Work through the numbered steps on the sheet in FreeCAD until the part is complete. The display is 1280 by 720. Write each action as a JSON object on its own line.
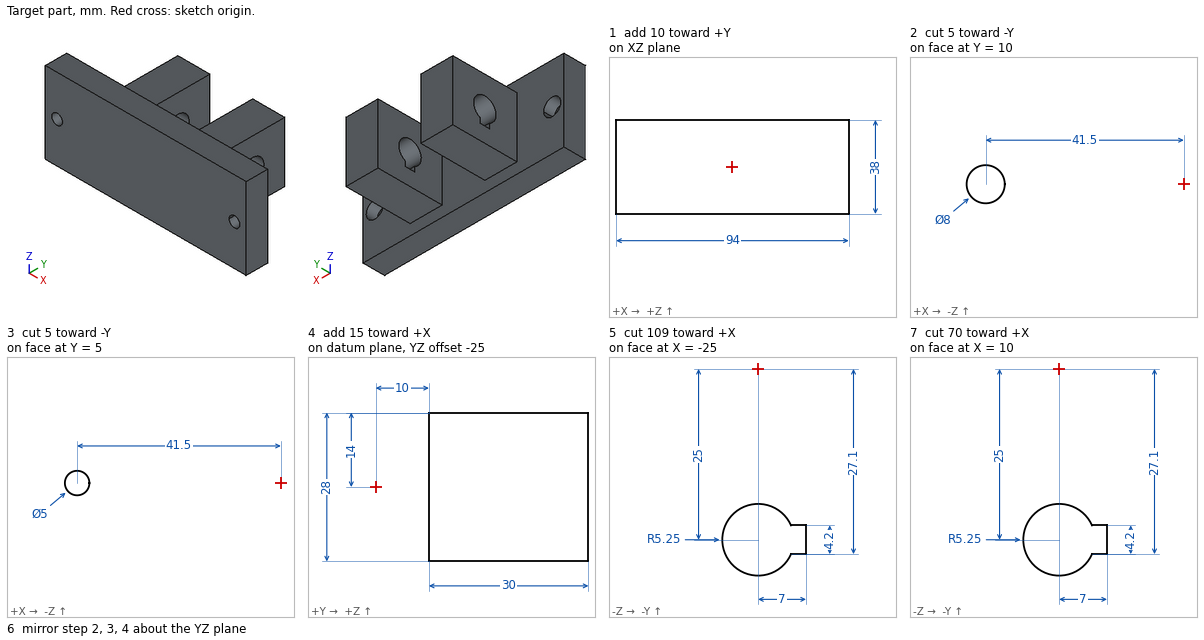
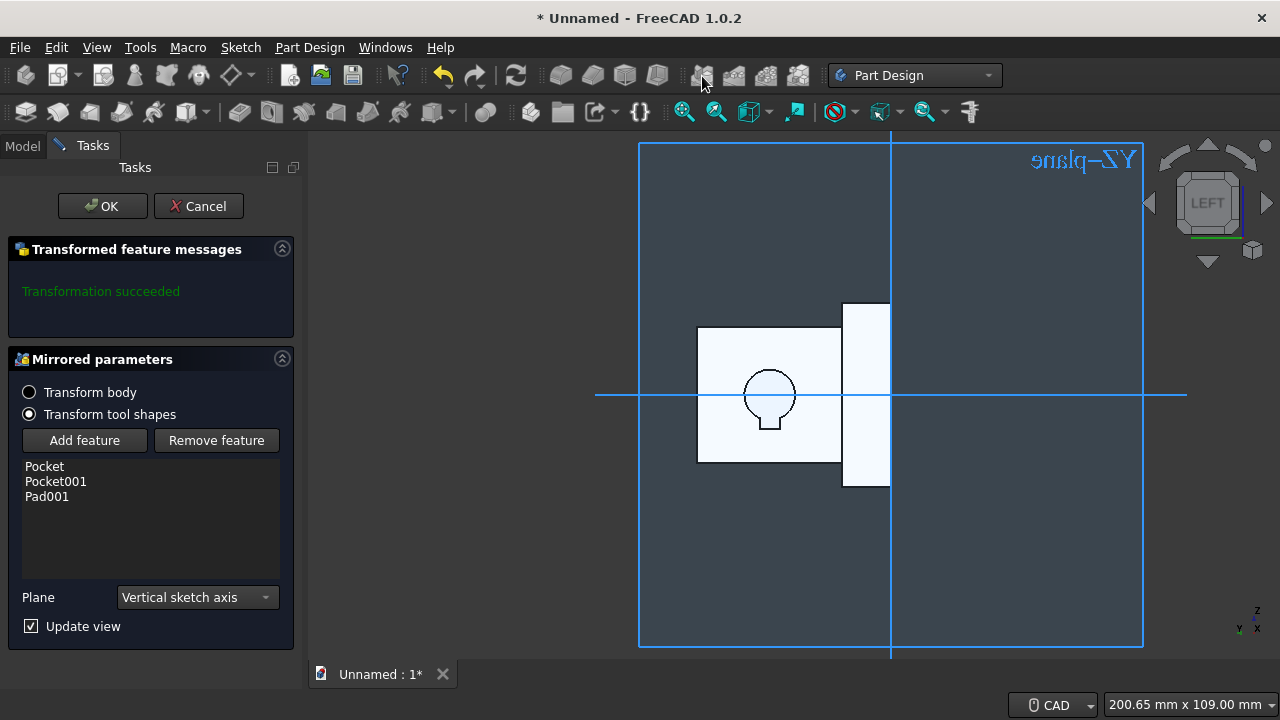
{"action": "left_click", "coordinate": [198, 598]}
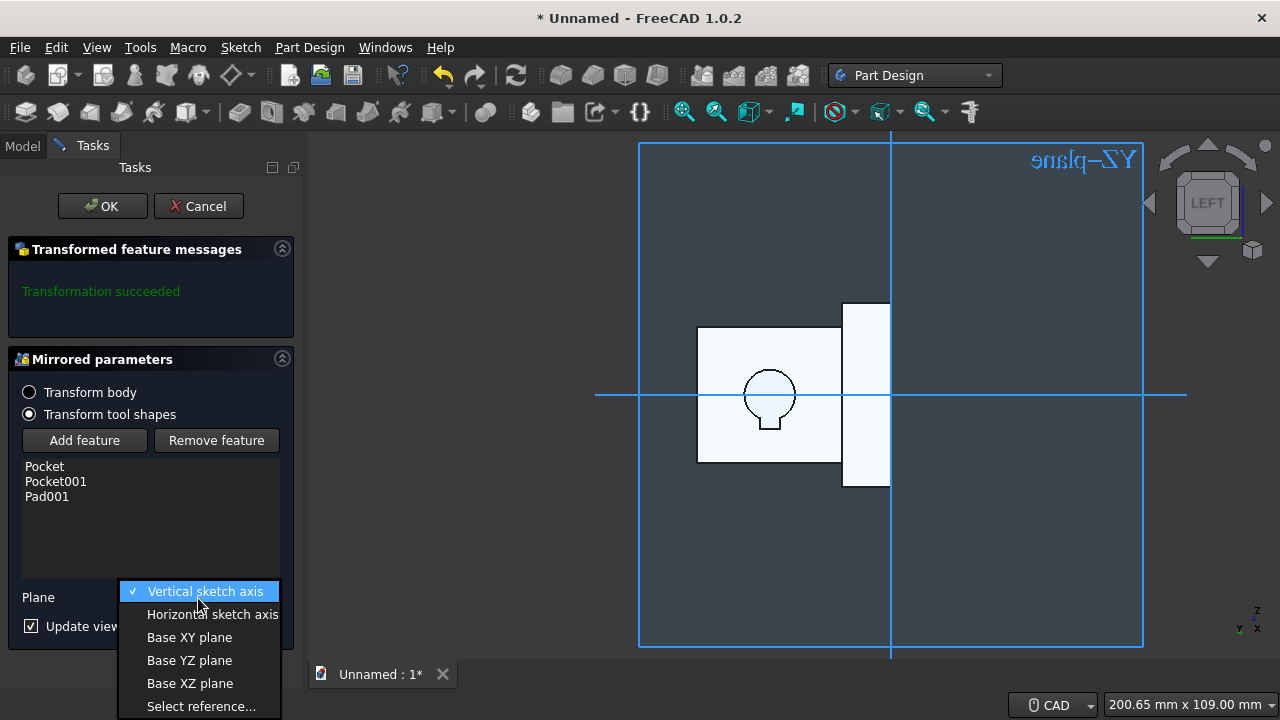
{"action": "left_click", "coordinate": [198, 660]}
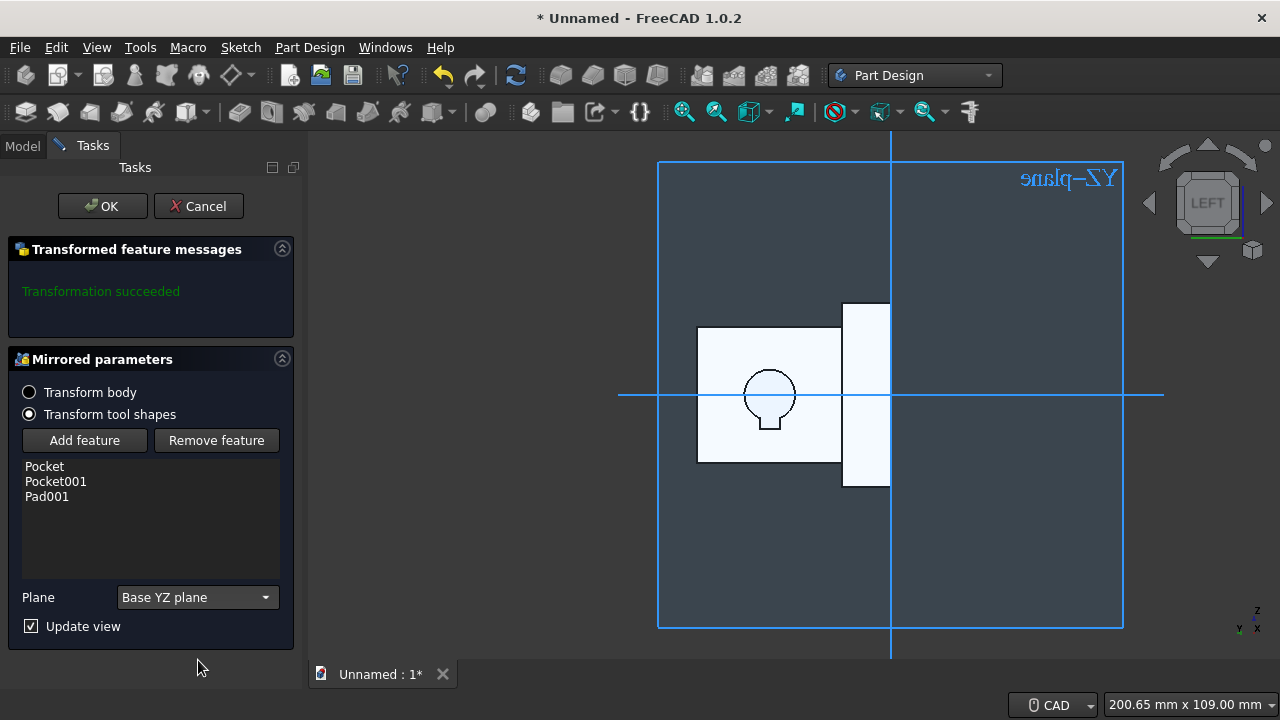
{"action": "left_click", "coordinate": [103, 206]}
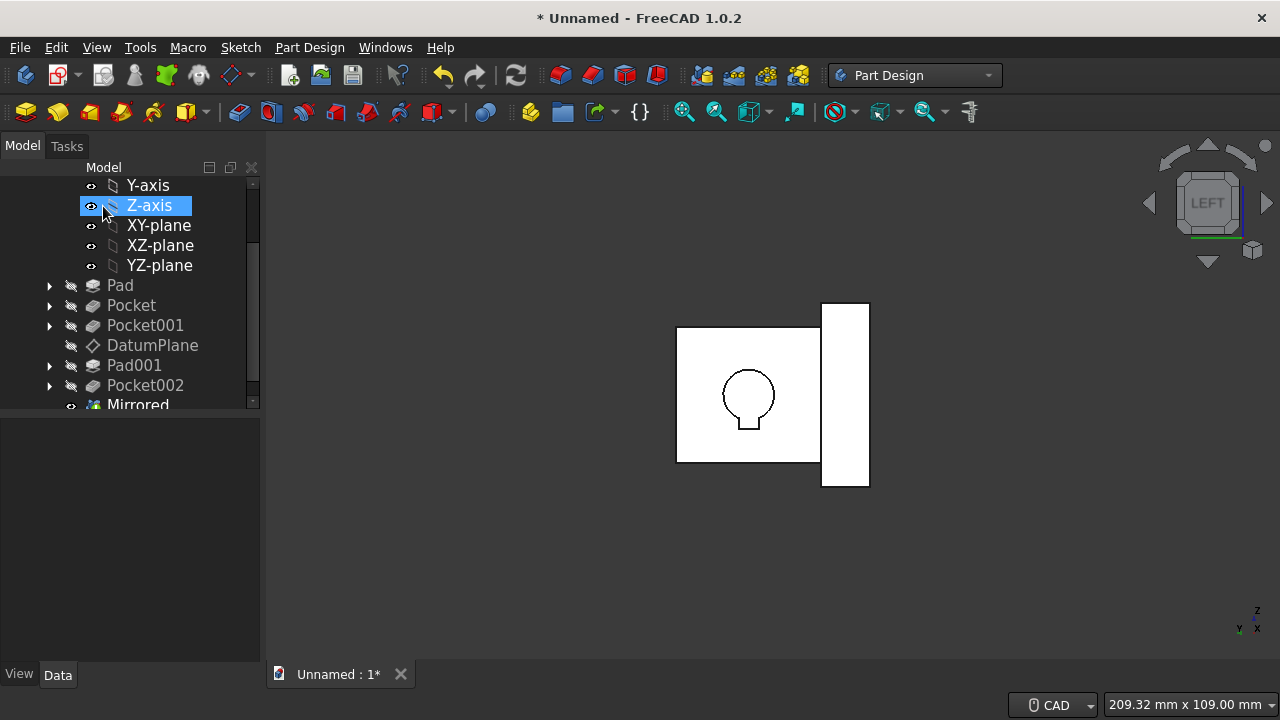
{"action": "left_click", "coordinate": [686, 112]}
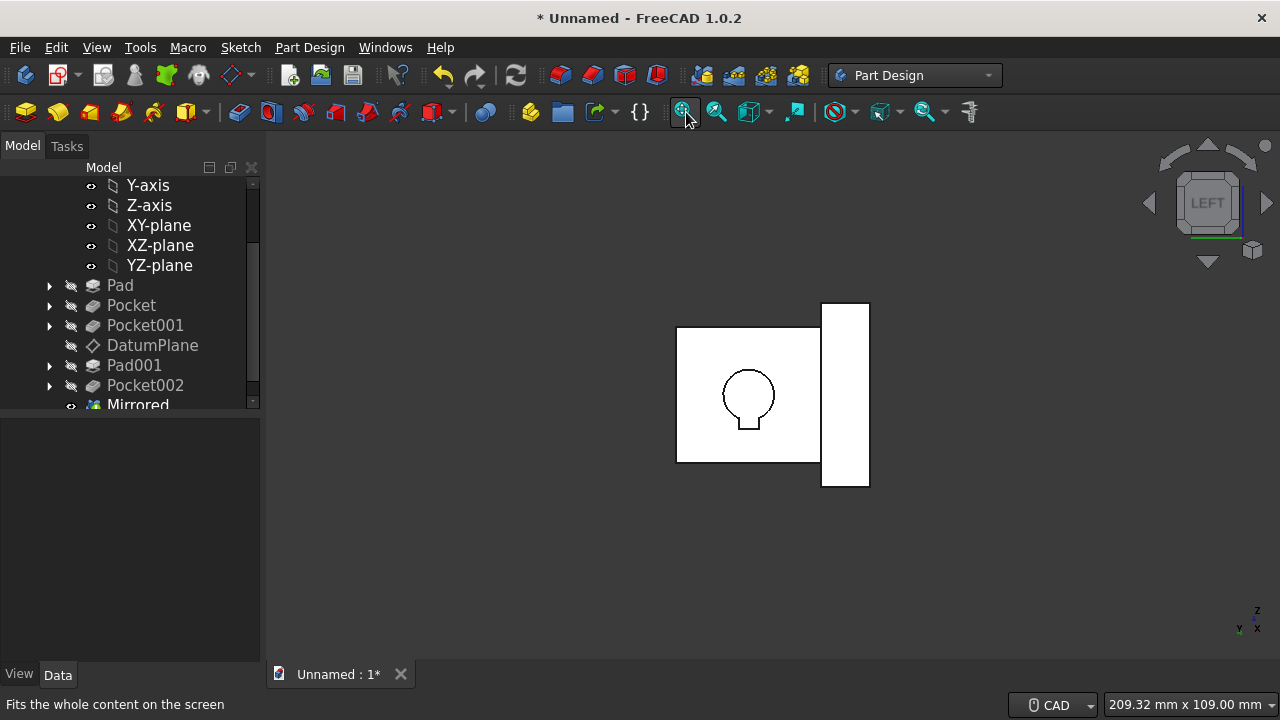
{"action": "left_click", "coordinate": [749, 394]}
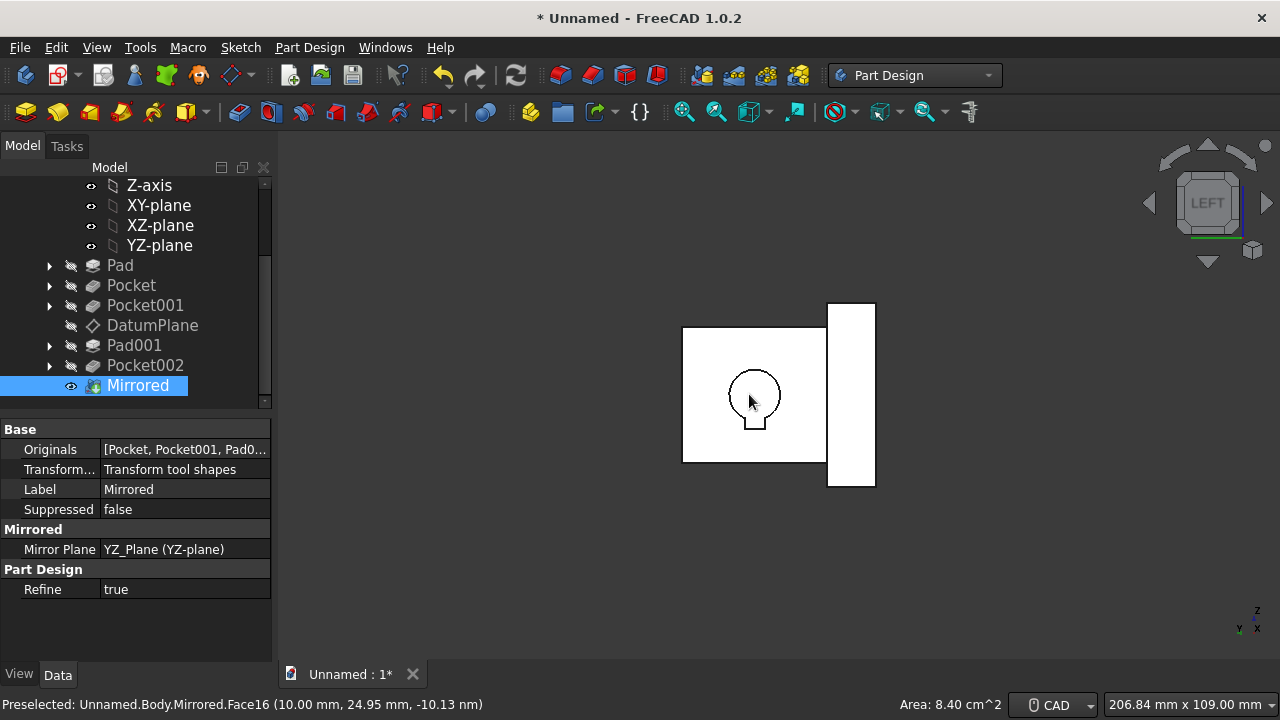
{"action": "left_click", "coordinate": [58, 76]}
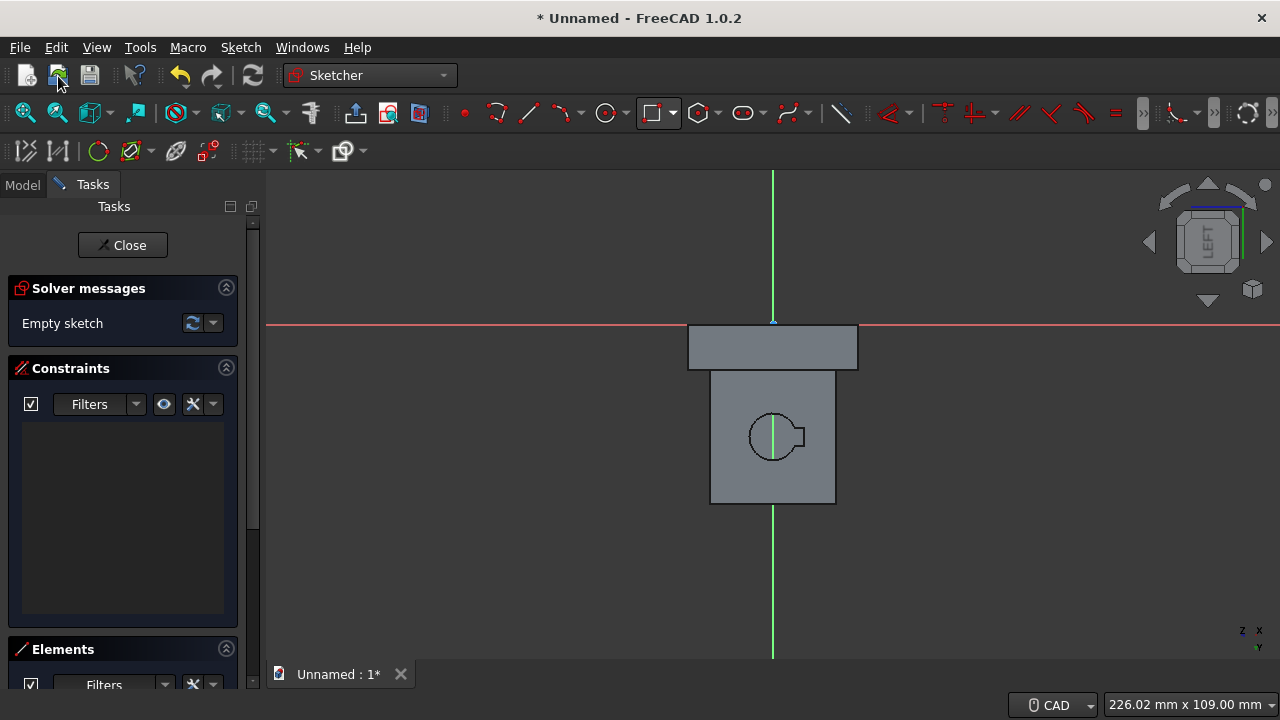
{"action": "scroll", "coordinate": [819, 369], "scroll_direction": "up", "scroll_amount": 5}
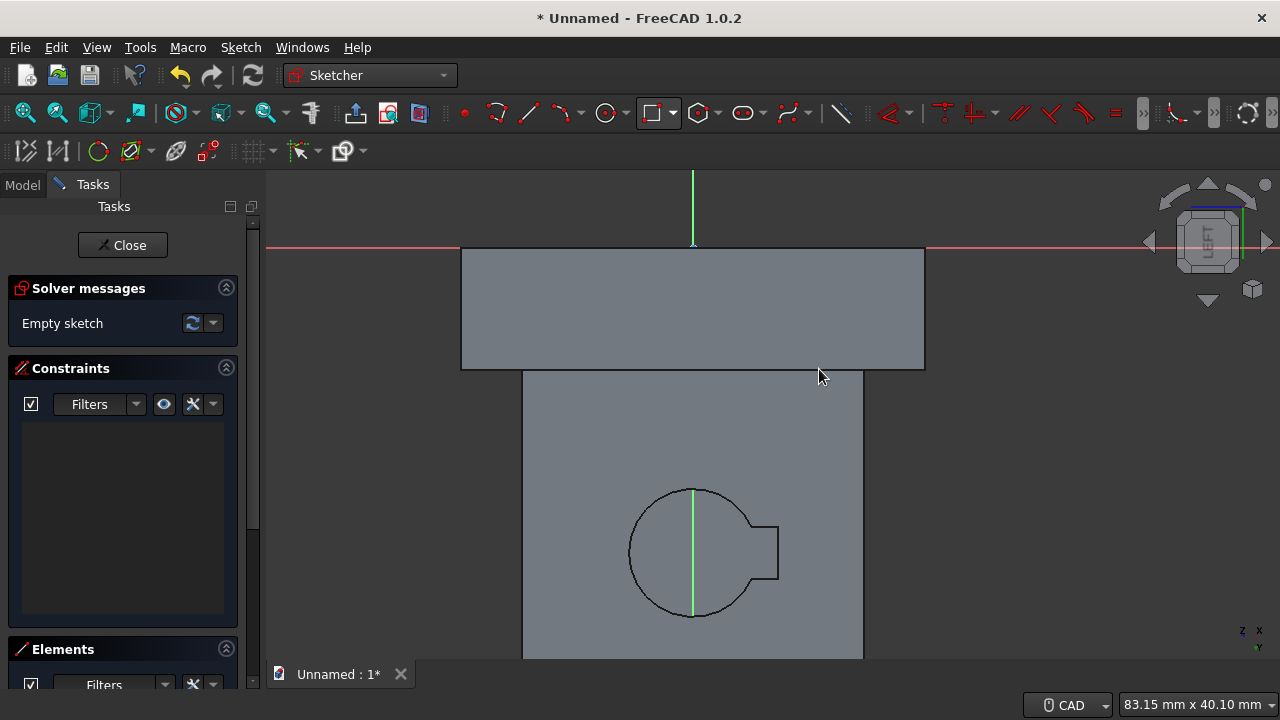
{"action": "left_click", "coordinate": [498, 114]}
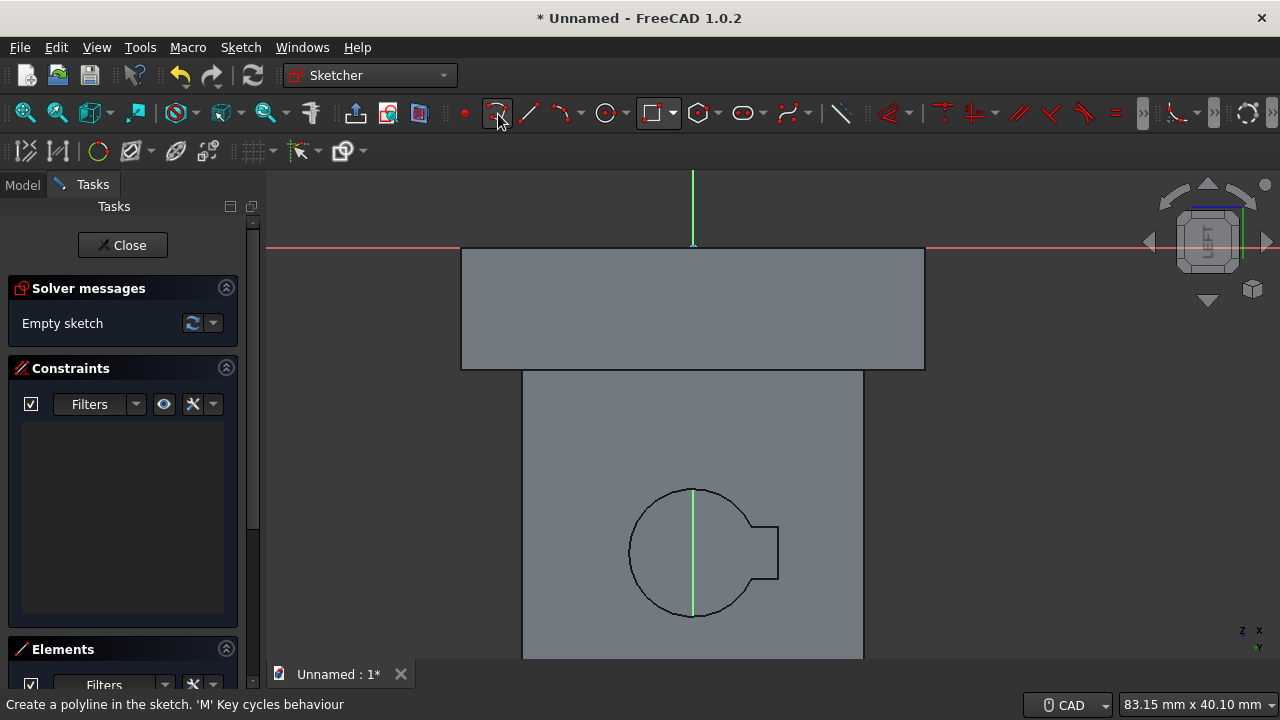
{"action": "left_click", "coordinate": [752, 579]}
{"action": "left_click", "coordinate": [778, 579]}
{"action": "left_click", "coordinate": [778, 527]}
{"action": "left_click", "coordinate": [752, 527]}
{"action": "right_click", "coordinate": [752, 527]}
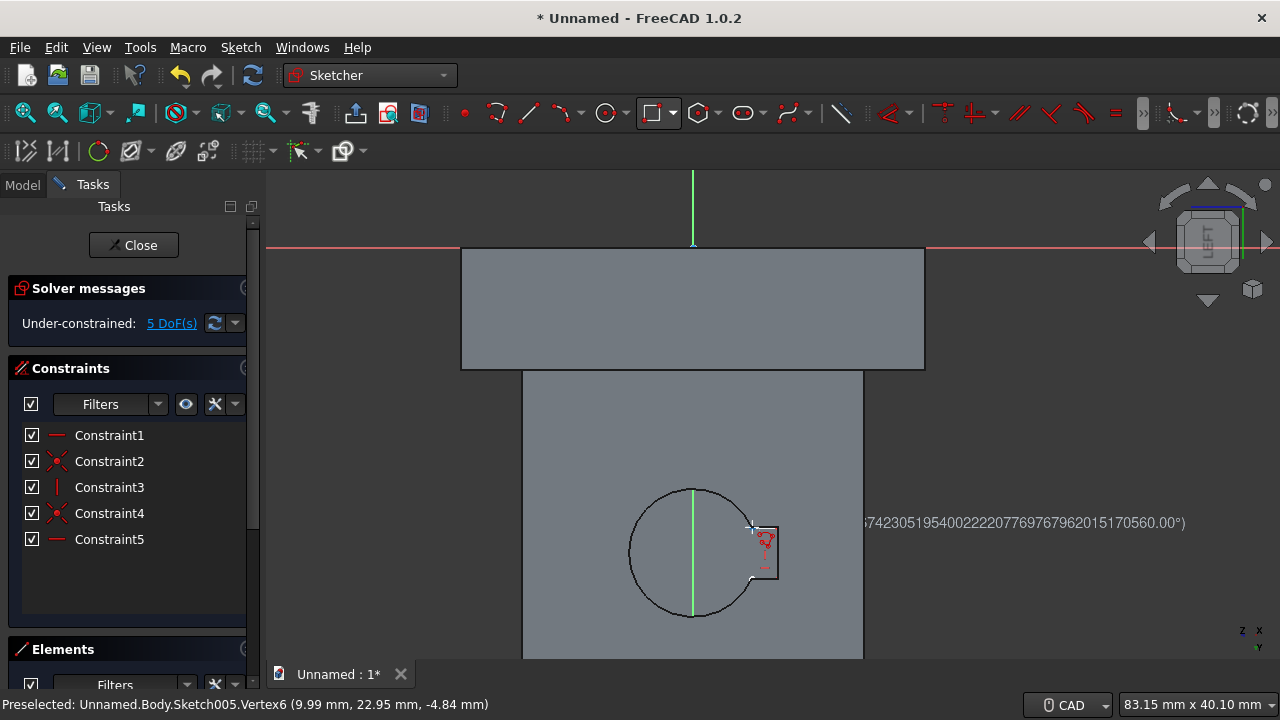
{"action": "left_click", "coordinate": [562, 114]}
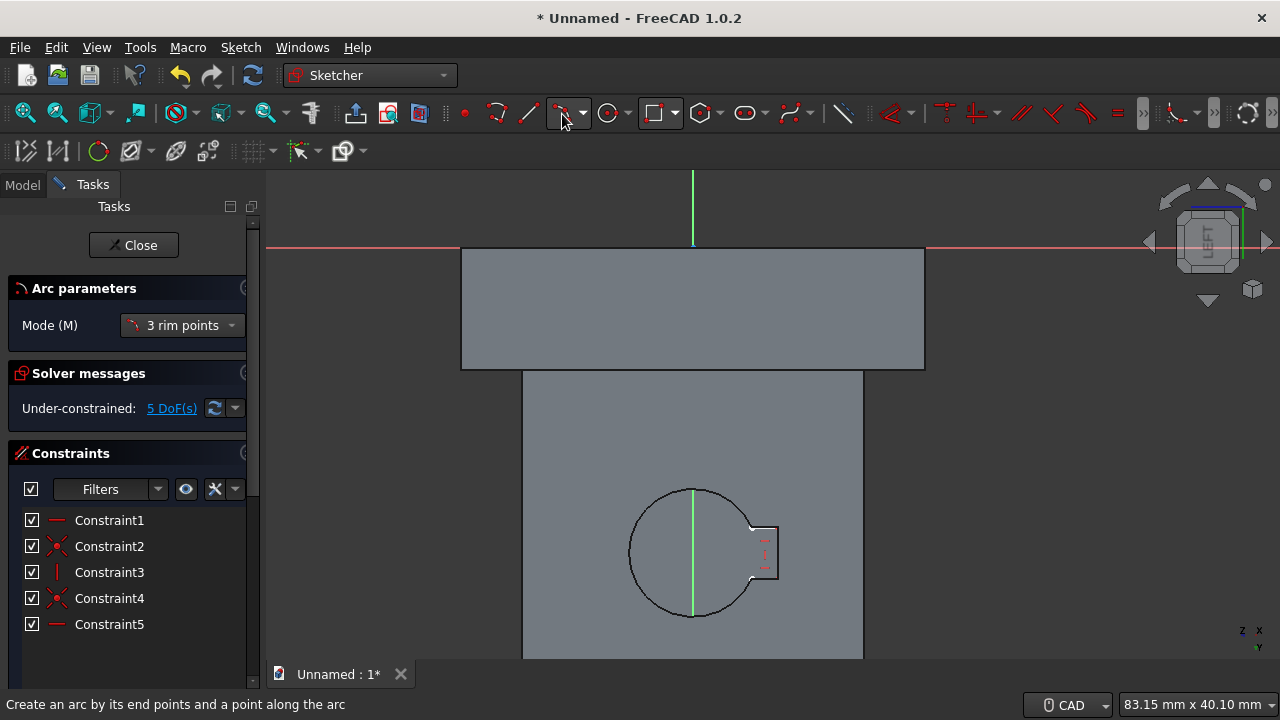
{"action": "left_click", "coordinate": [752, 528]}
{"action": "left_click", "coordinate": [752, 580]}
{"action": "left_click", "coordinate": [629, 553]}
{"action": "key", "text": "Escape"}